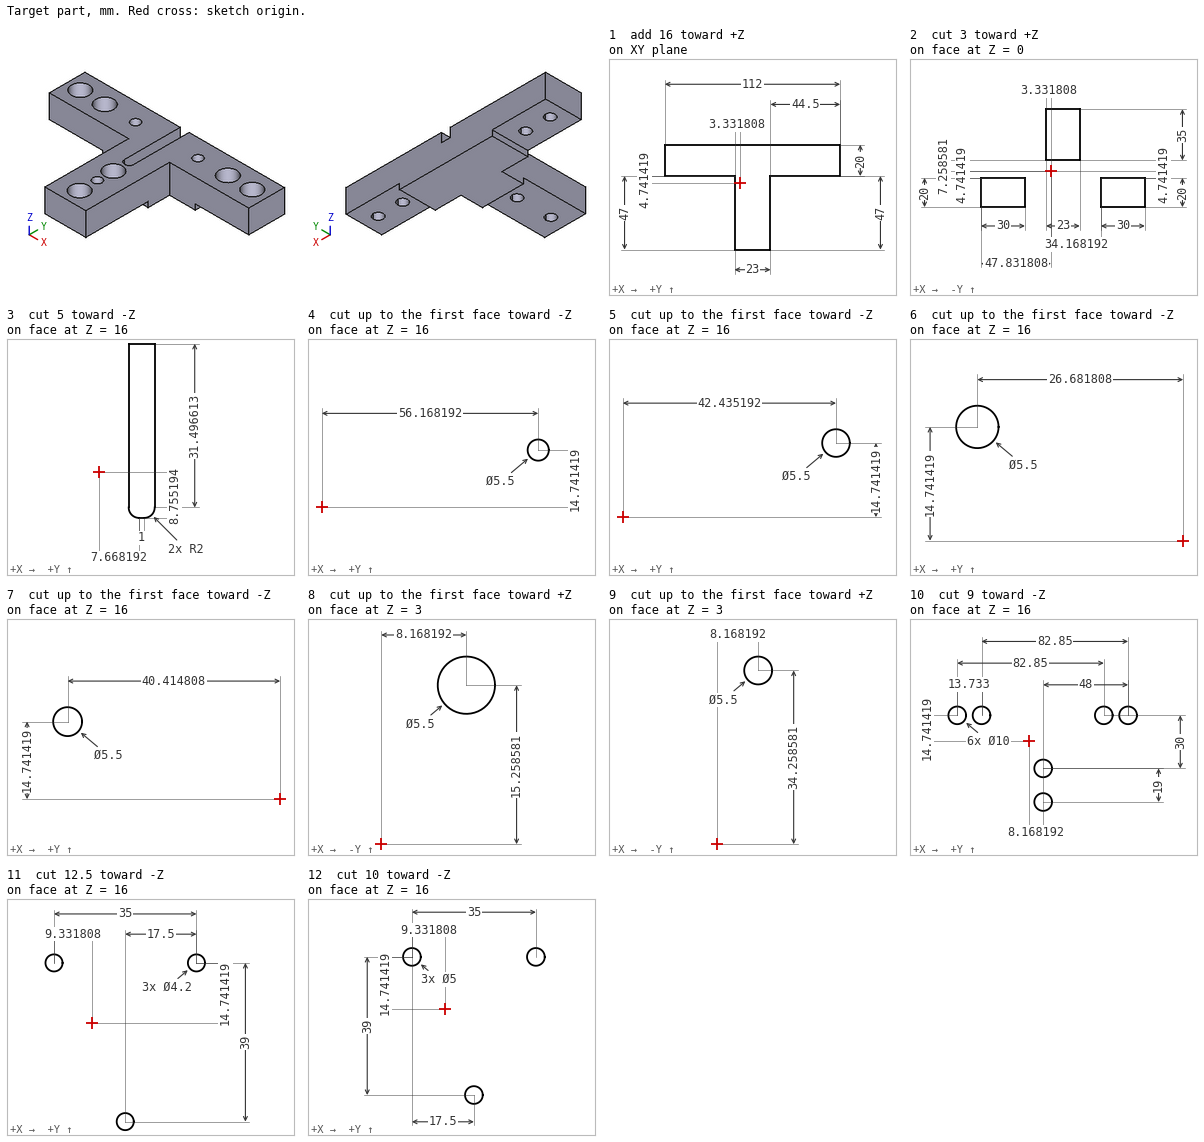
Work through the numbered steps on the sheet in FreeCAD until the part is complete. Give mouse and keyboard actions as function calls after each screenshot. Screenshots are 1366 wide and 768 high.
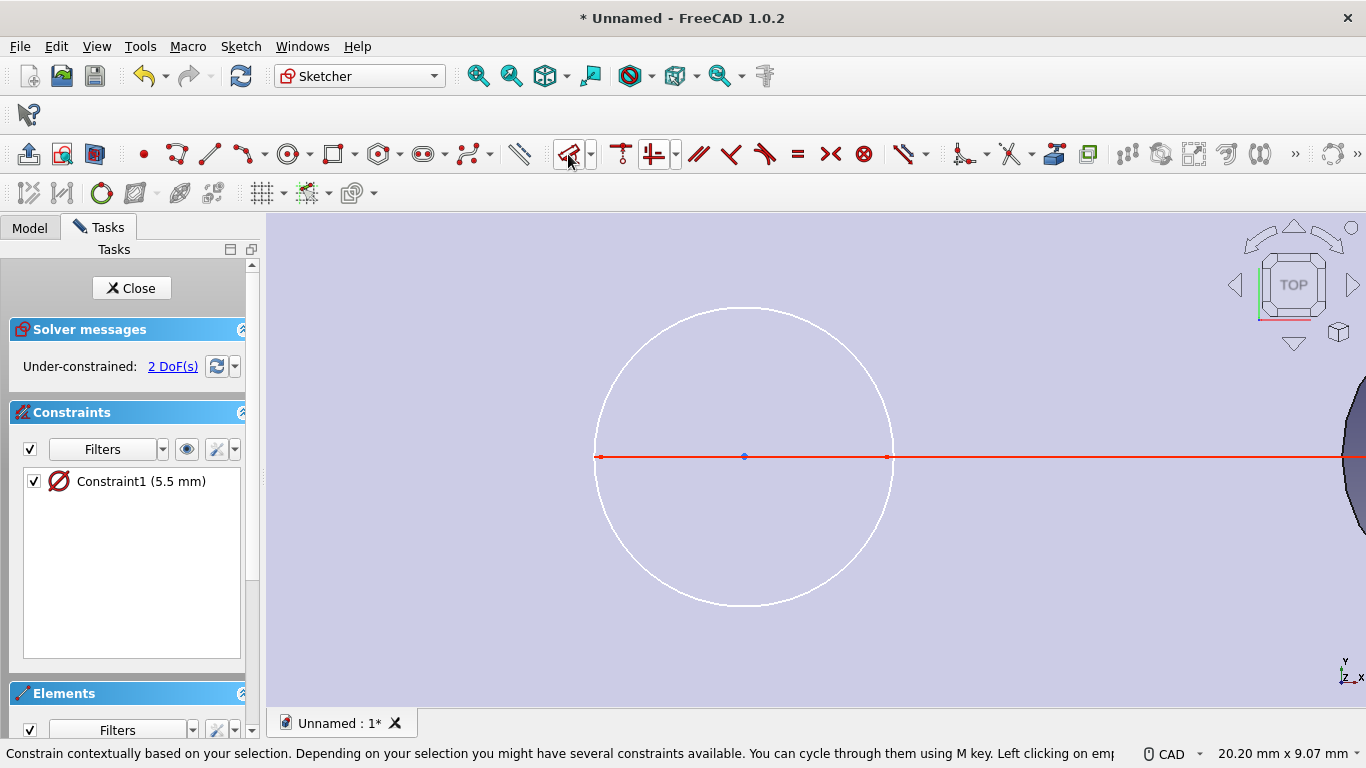
click(744, 457)
click(519, 423)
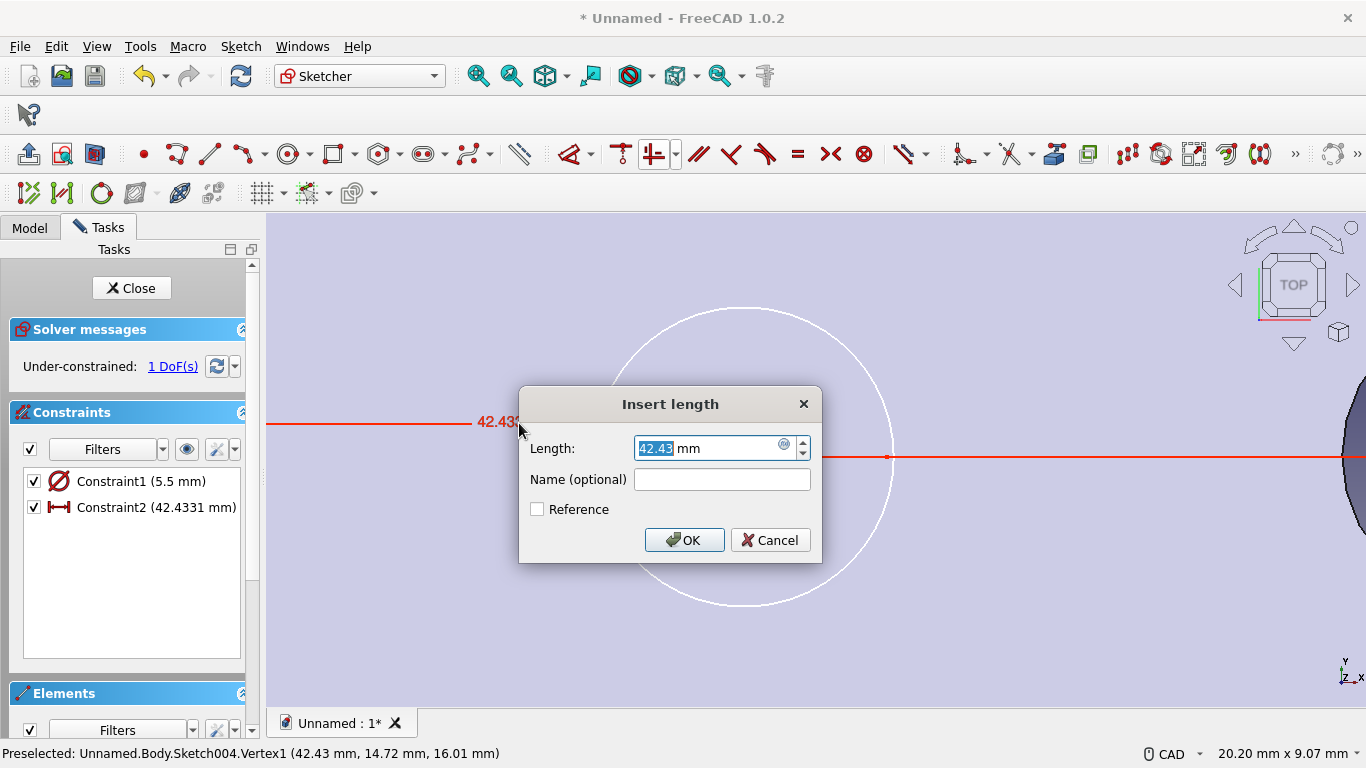
text(42.435192)
key(Return)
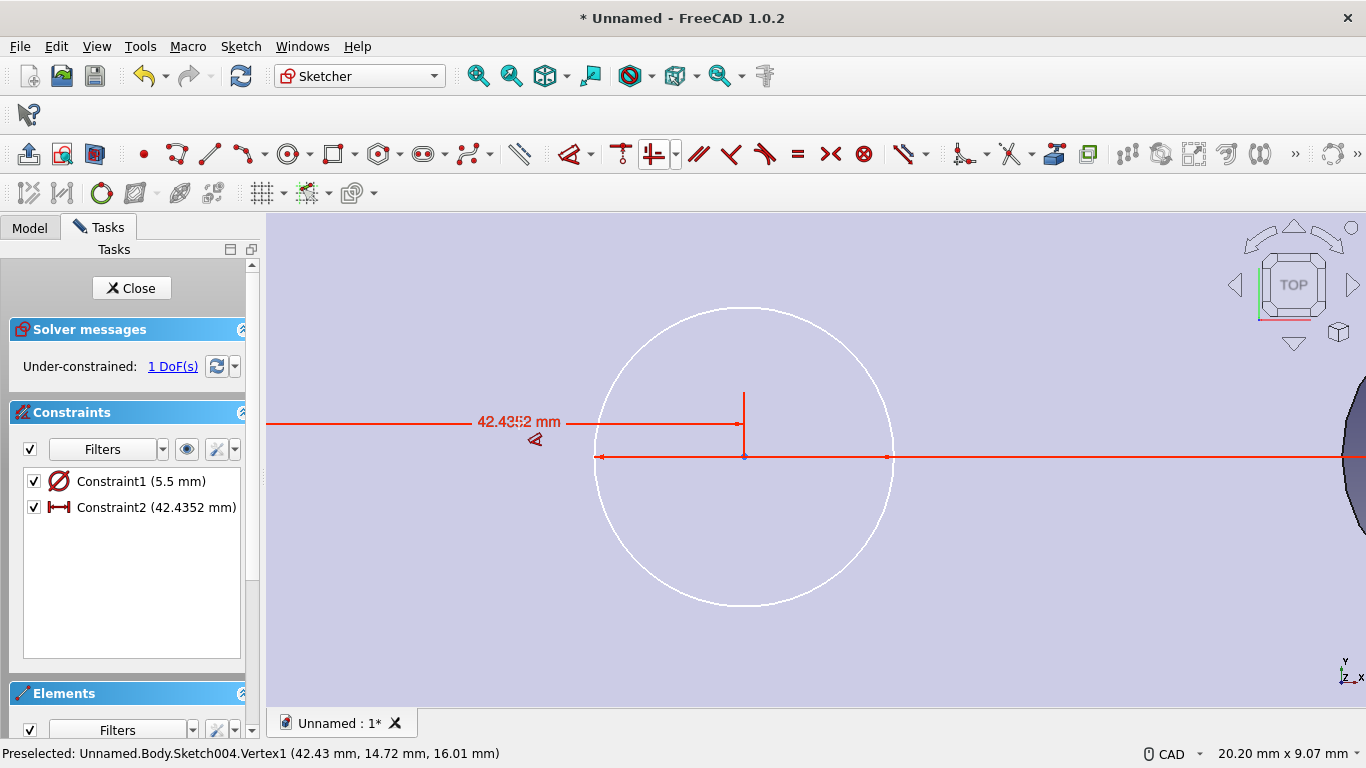
click(744, 457)
click(778, 568)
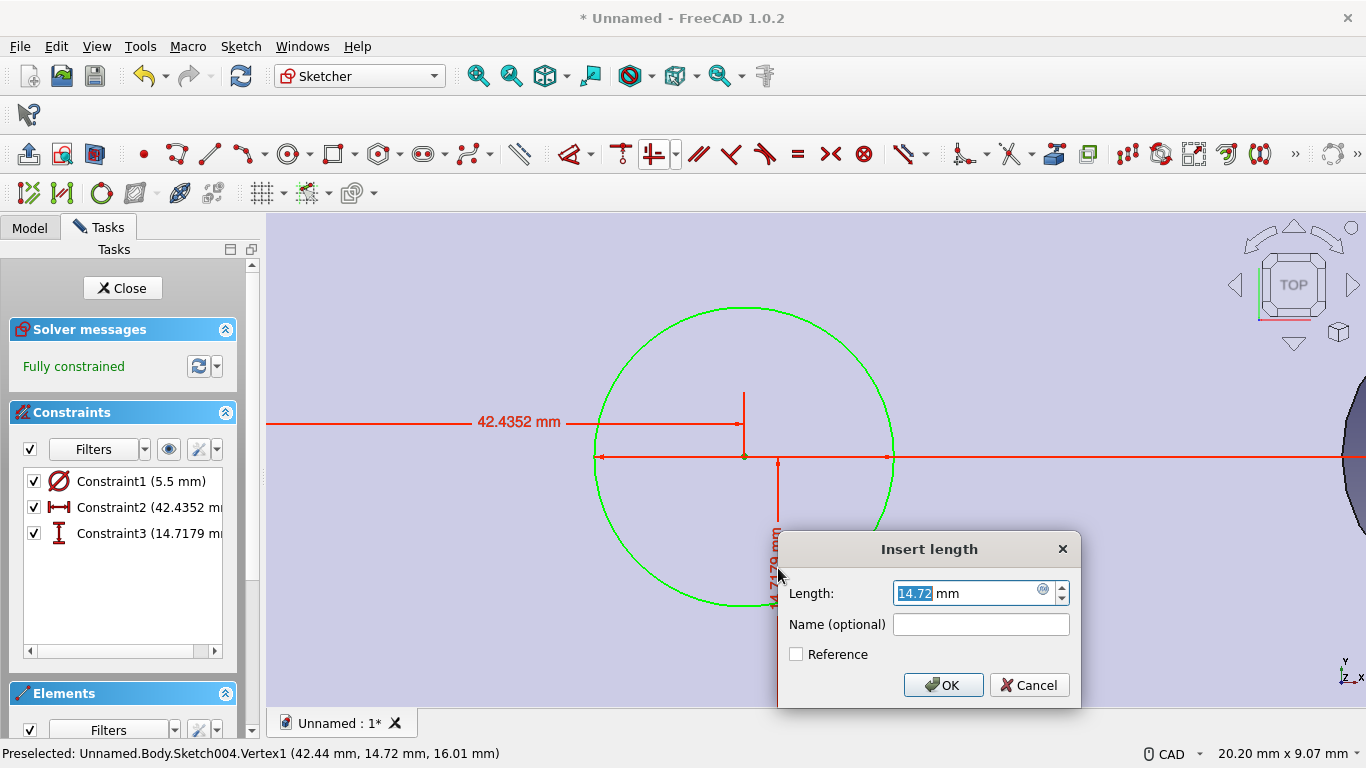
text(14.741419)
key(Return)
key(Escape)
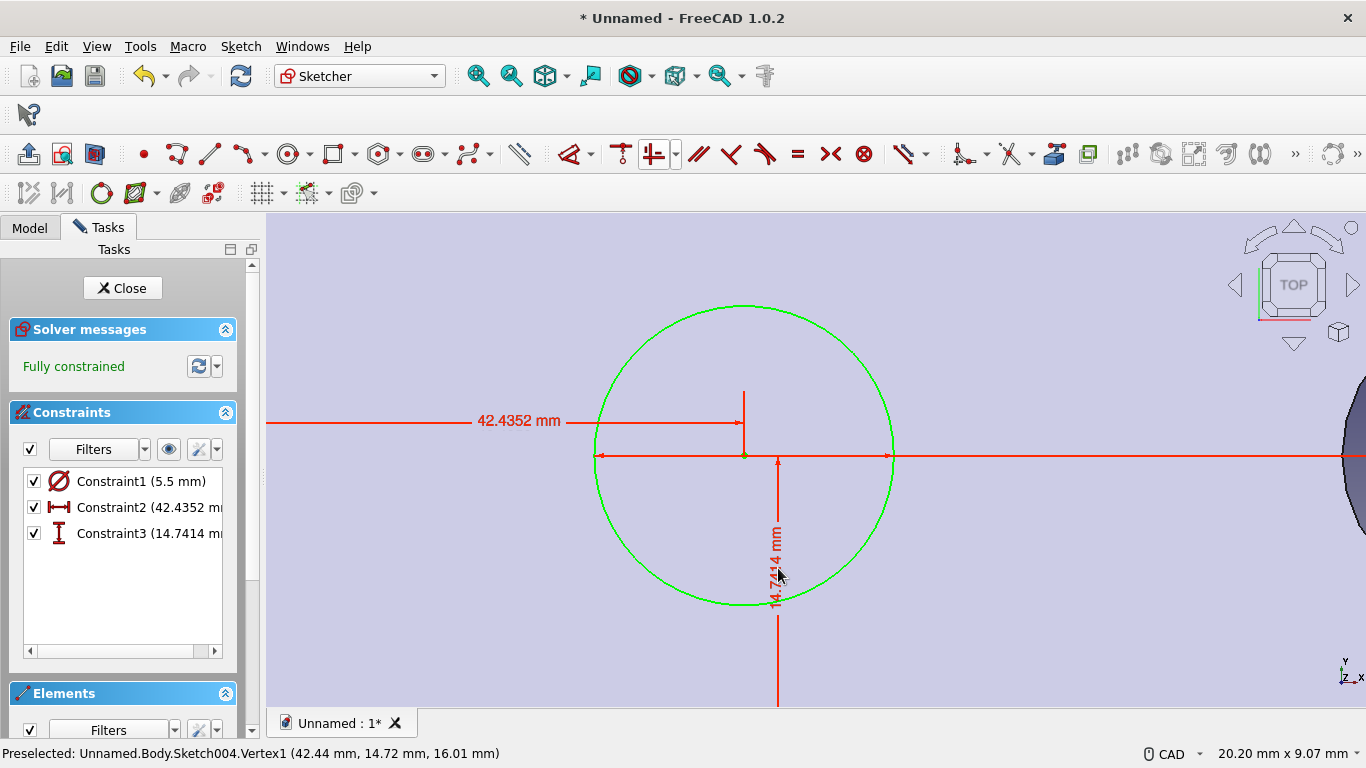
click(123, 288)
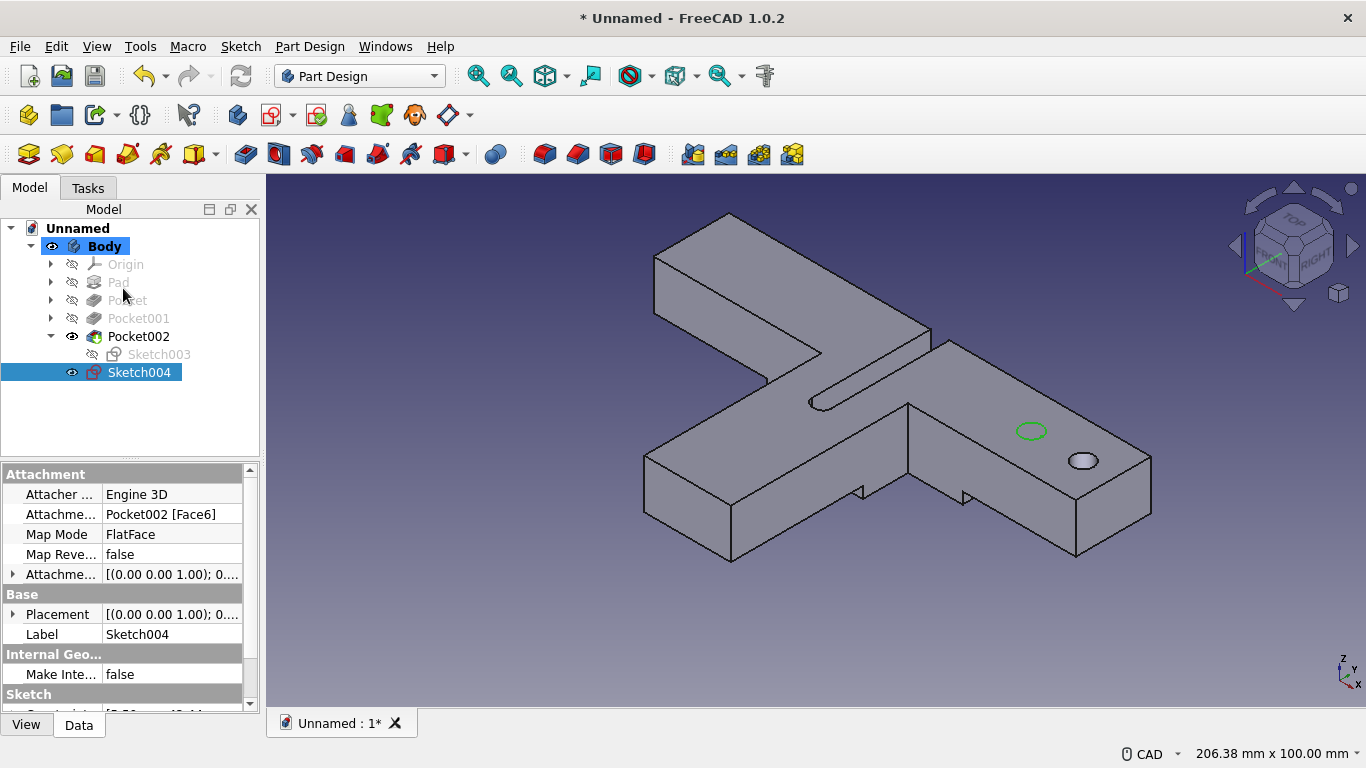
click(246, 154)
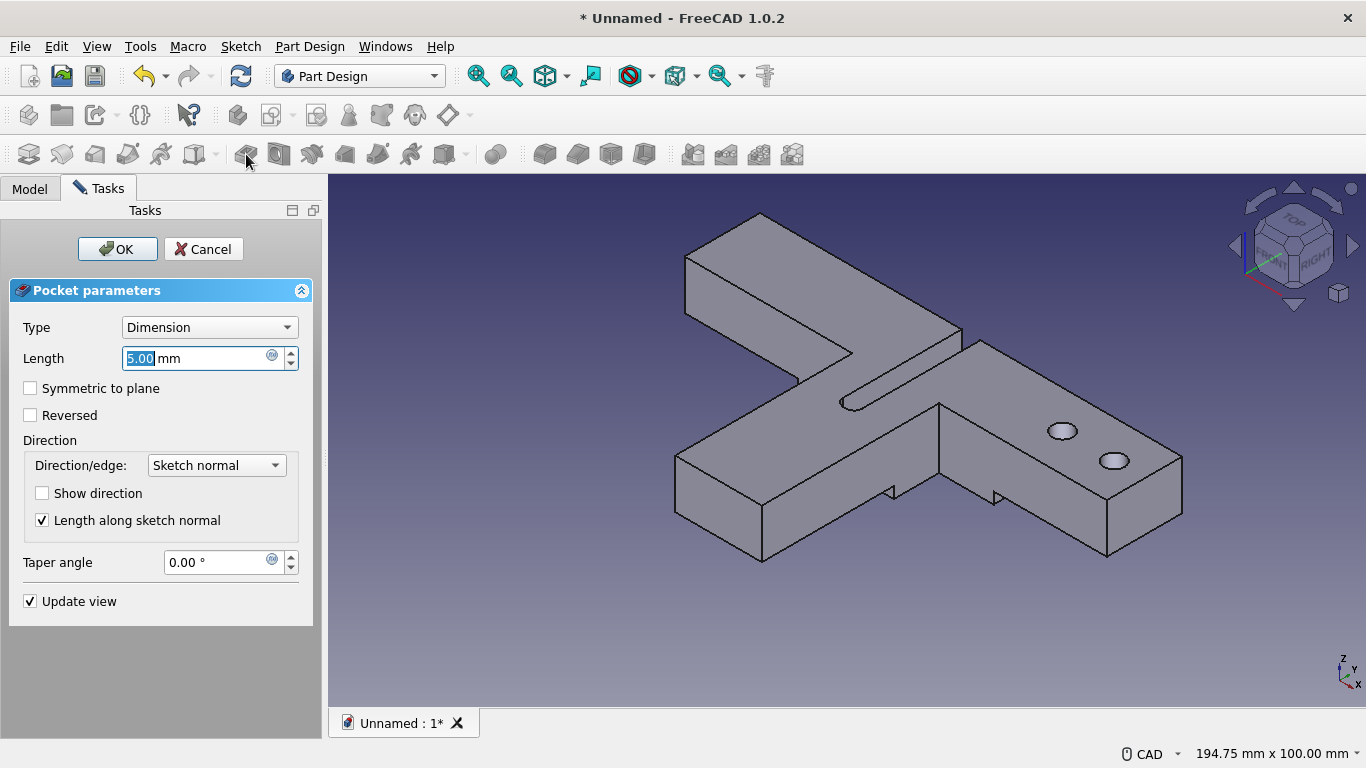
click(210, 328)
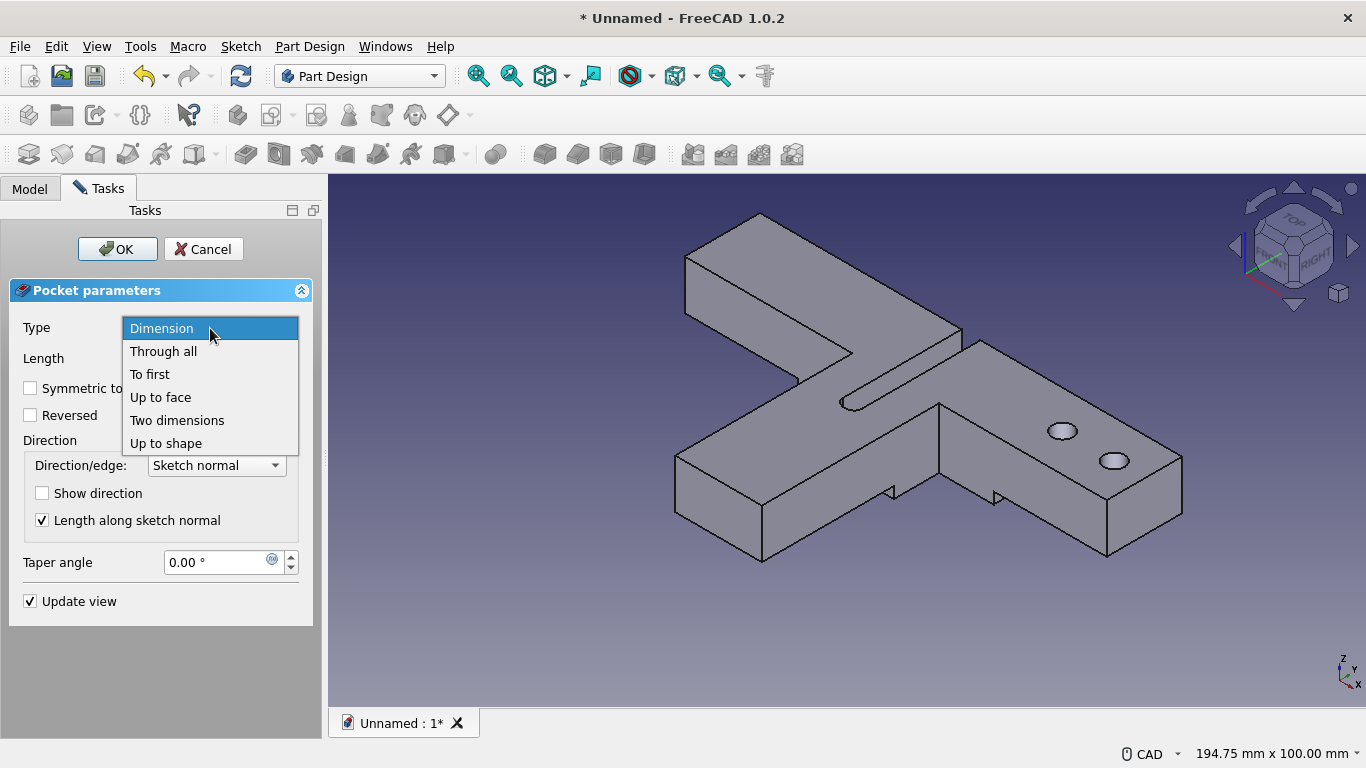
click(208, 374)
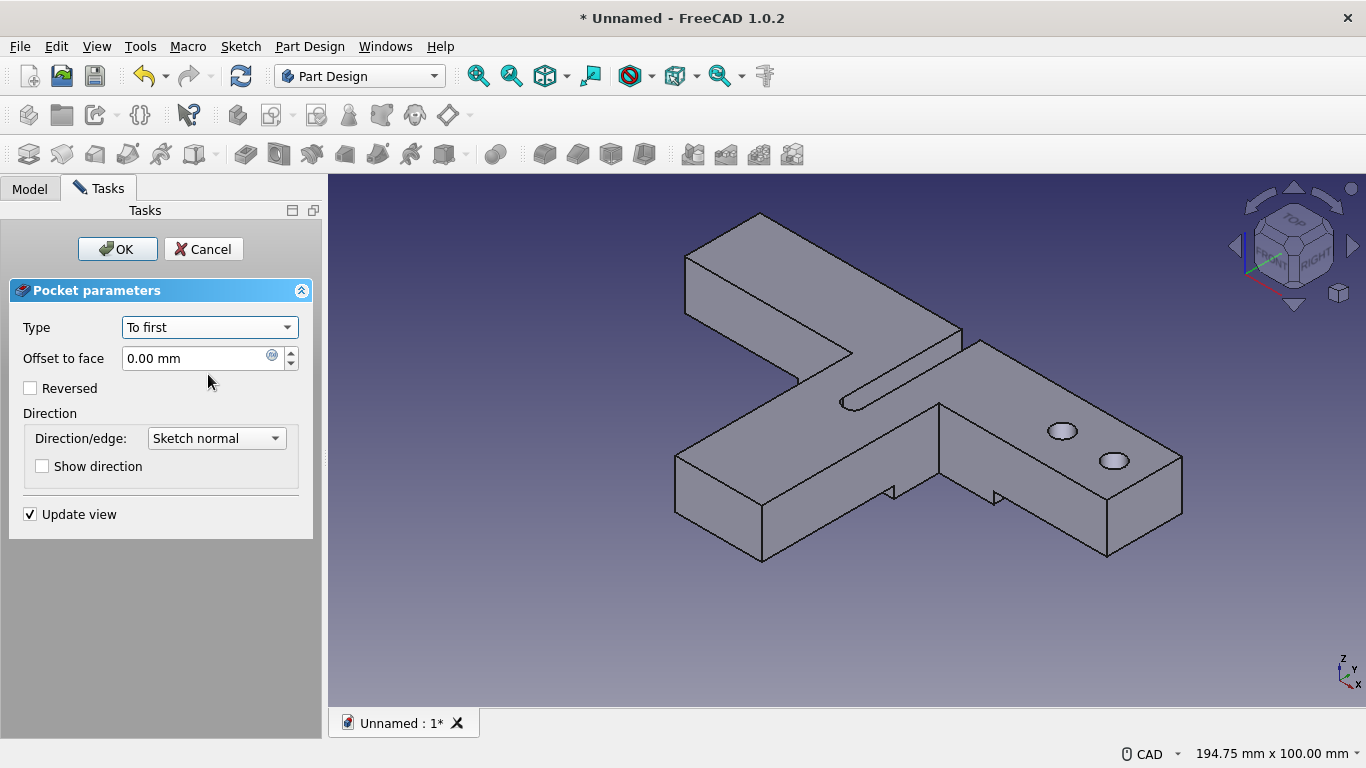
click(118, 249)